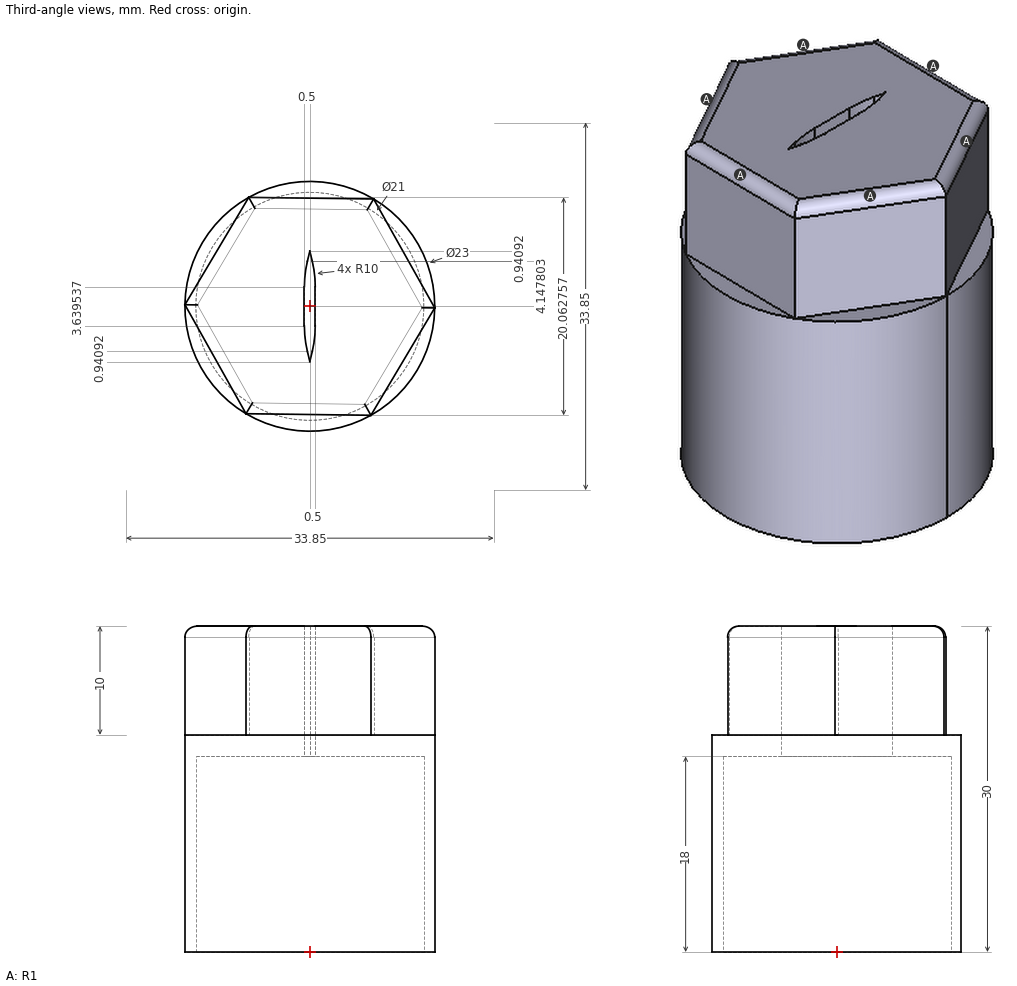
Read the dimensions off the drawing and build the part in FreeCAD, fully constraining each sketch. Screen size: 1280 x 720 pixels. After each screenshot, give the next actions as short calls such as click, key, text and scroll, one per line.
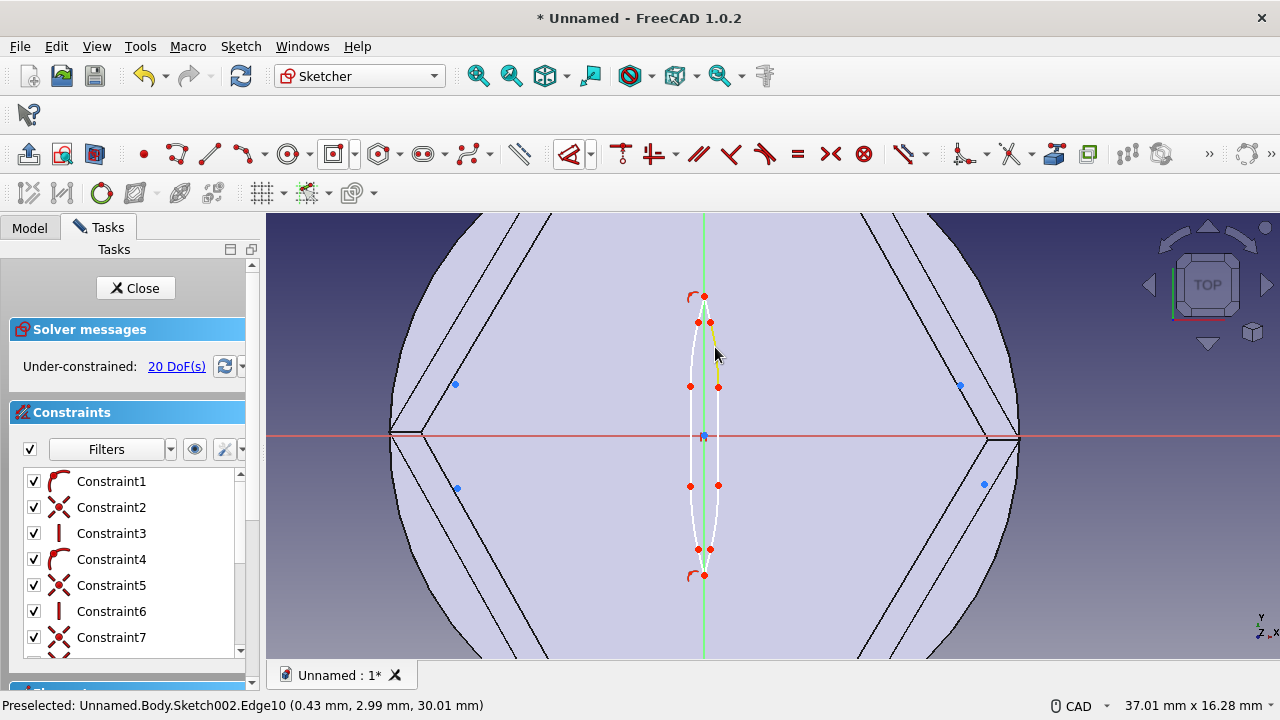
scroll(709, 315, up, 6)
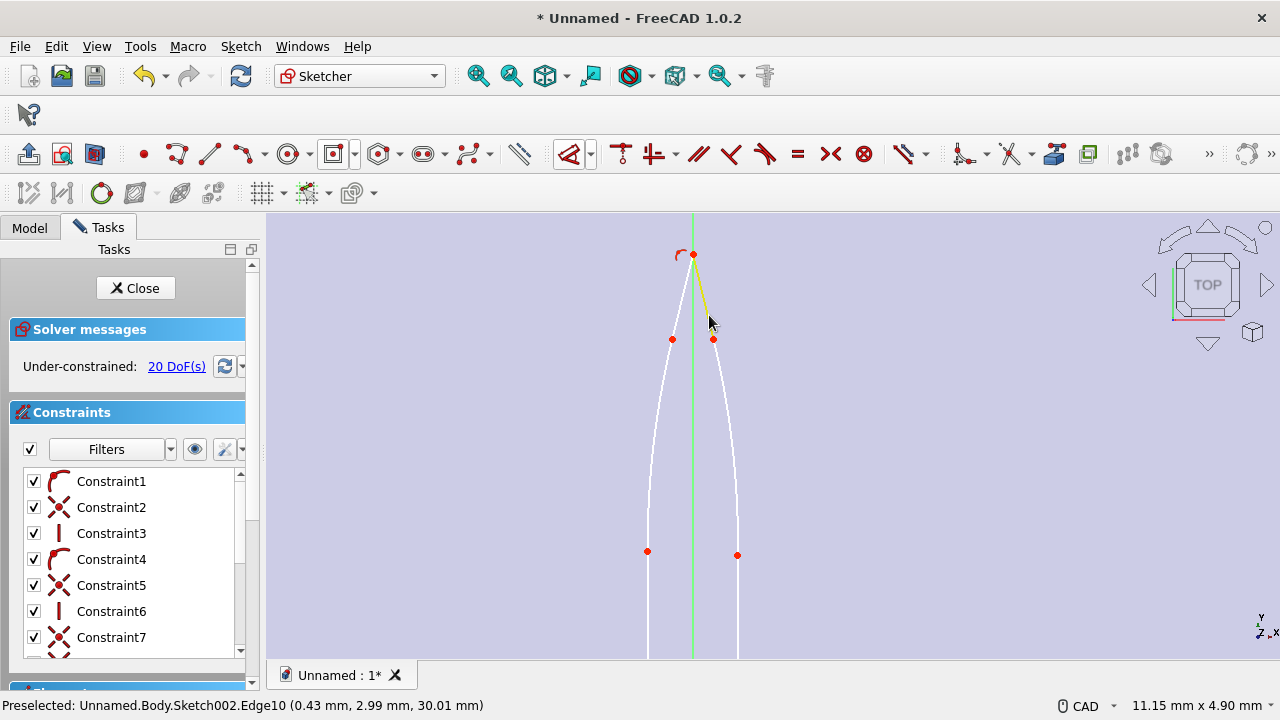
click(707, 314)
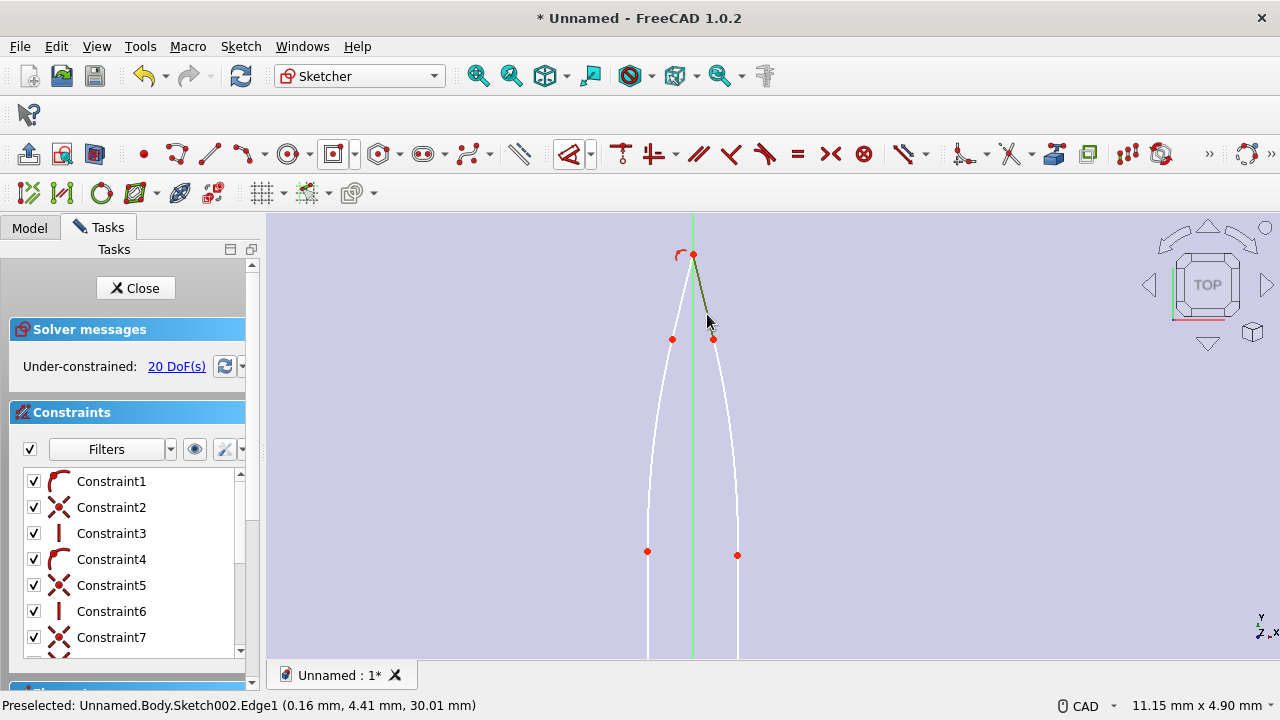
click(736, 490)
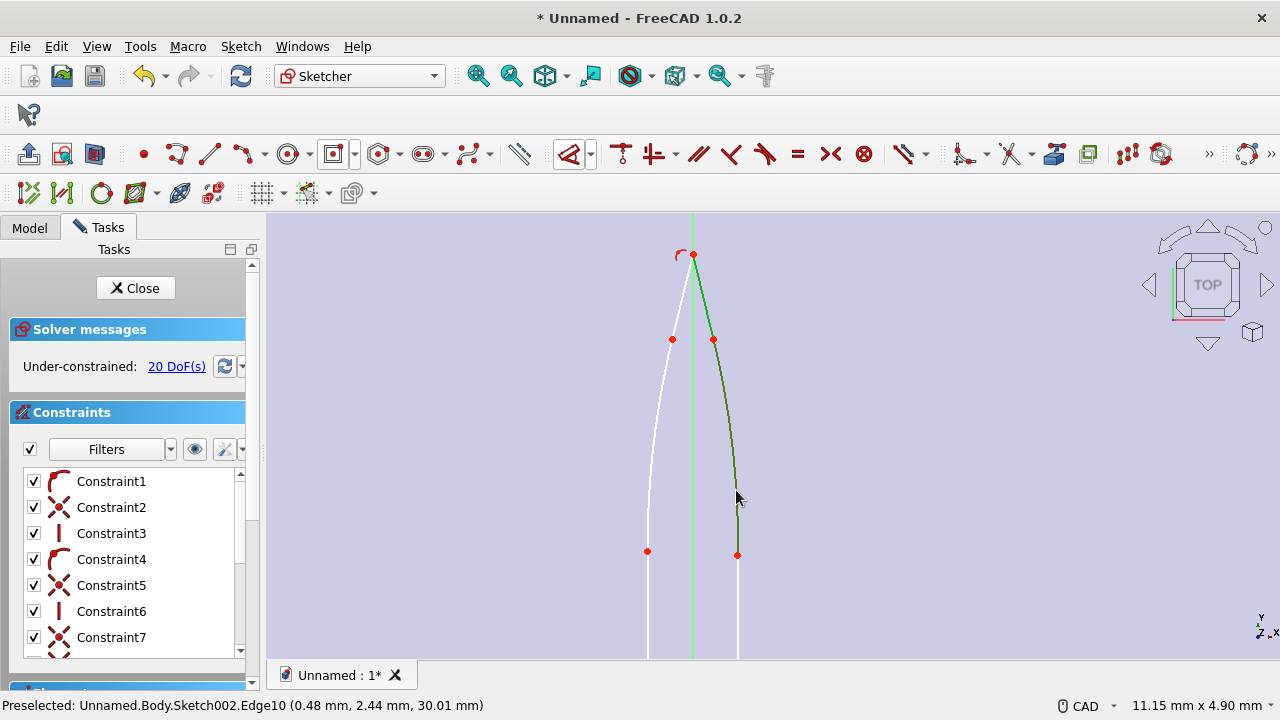
click(765, 154)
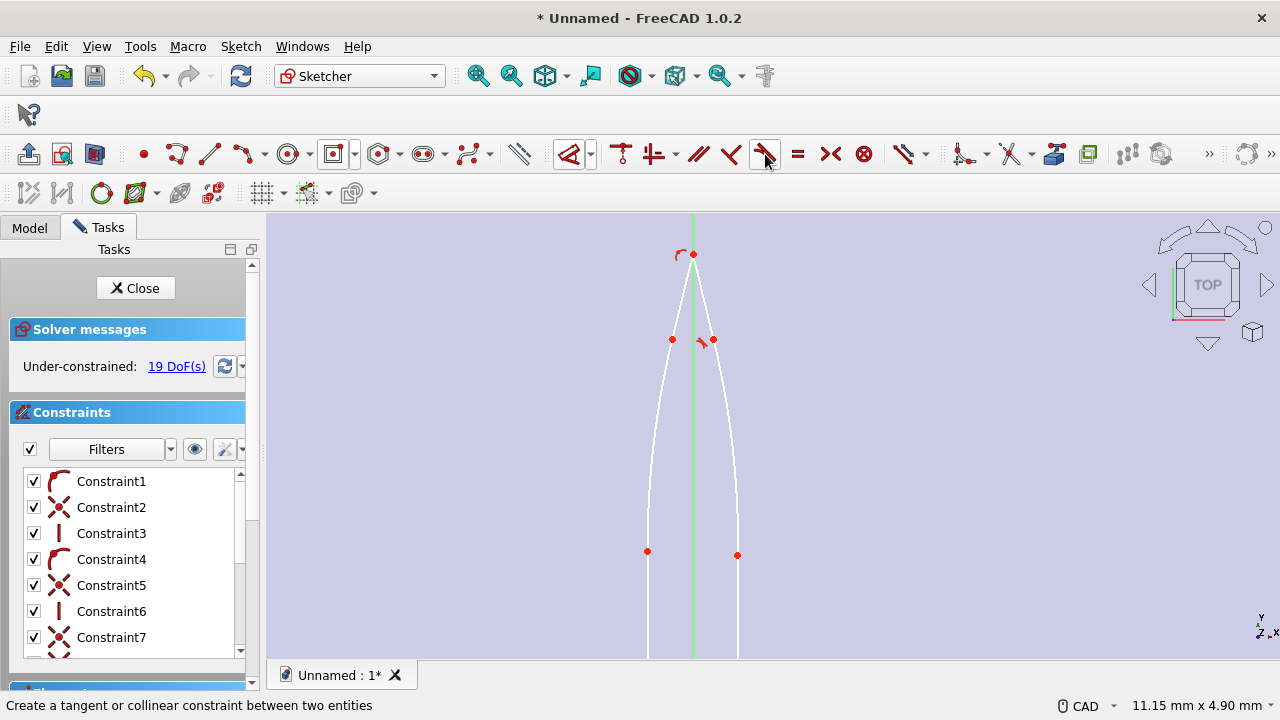
click(678, 314)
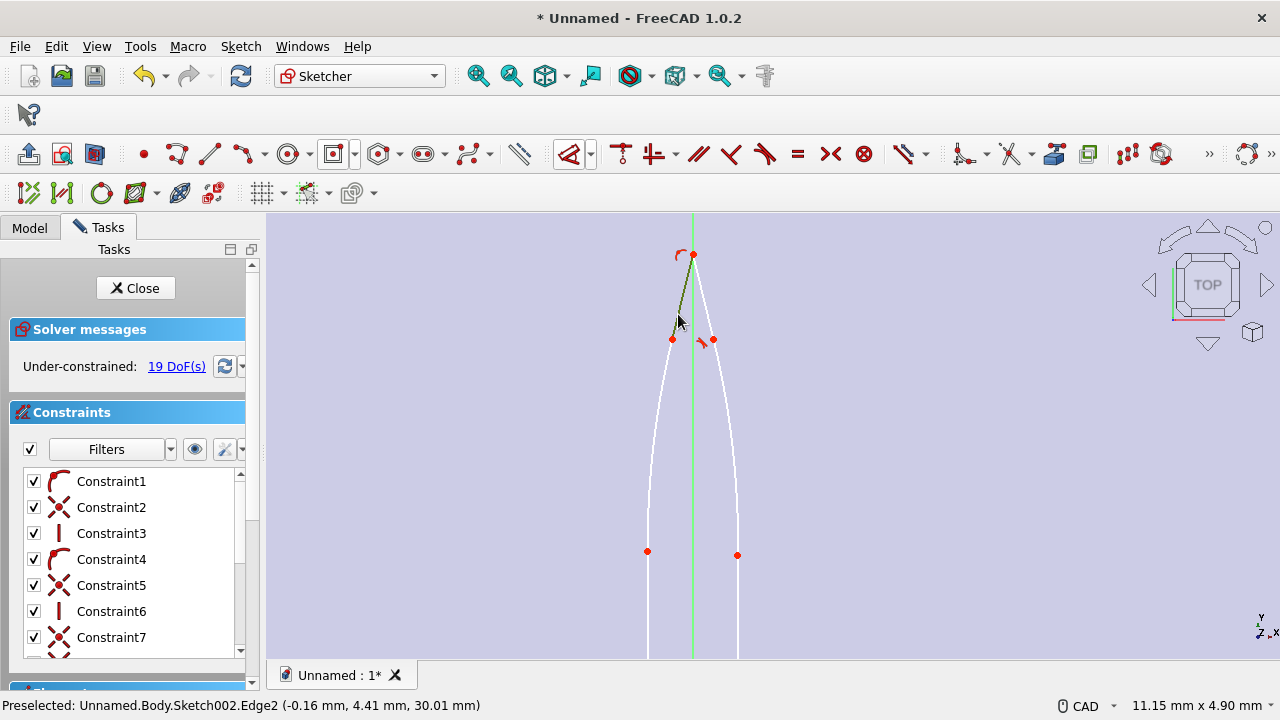
click(659, 403)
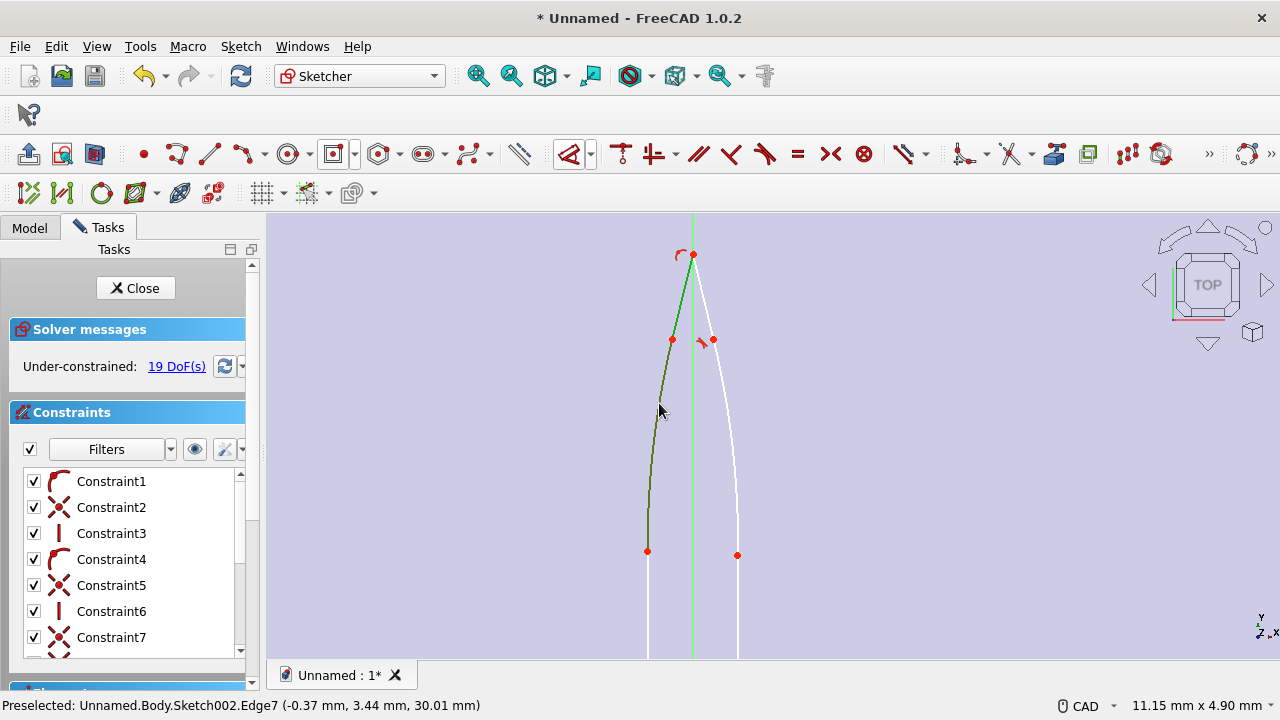
click(765, 154)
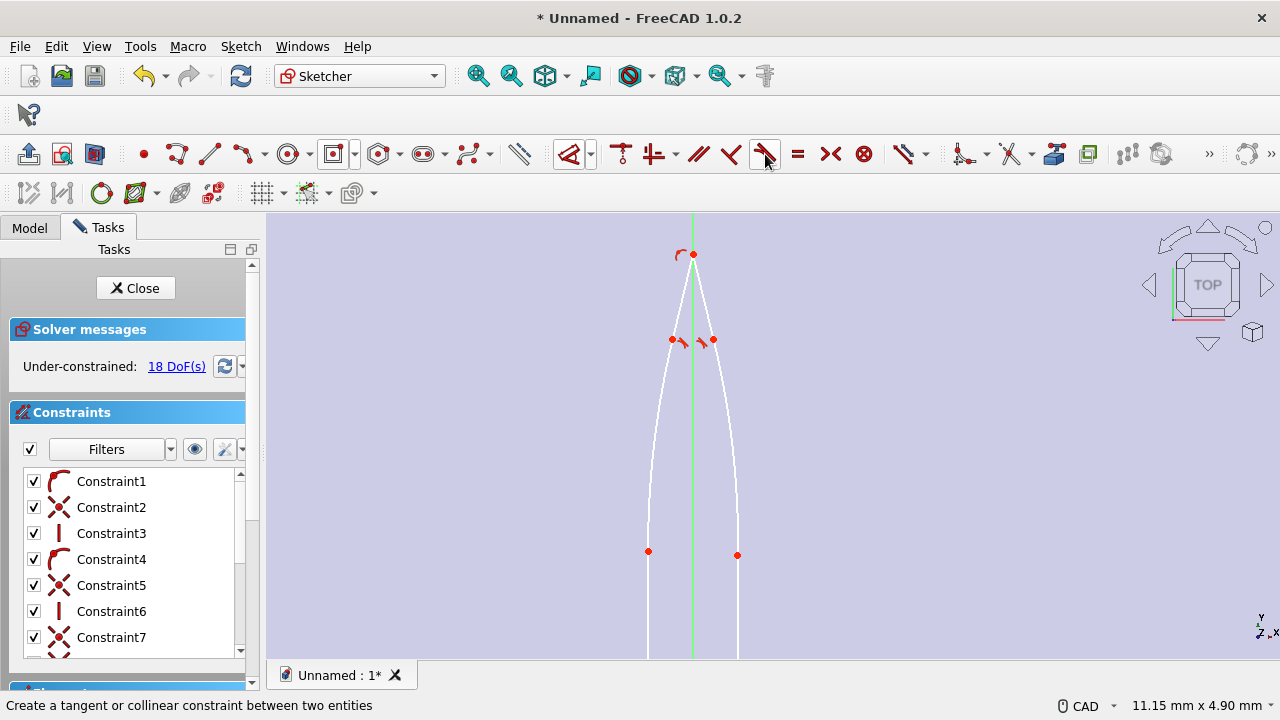
click(648, 618)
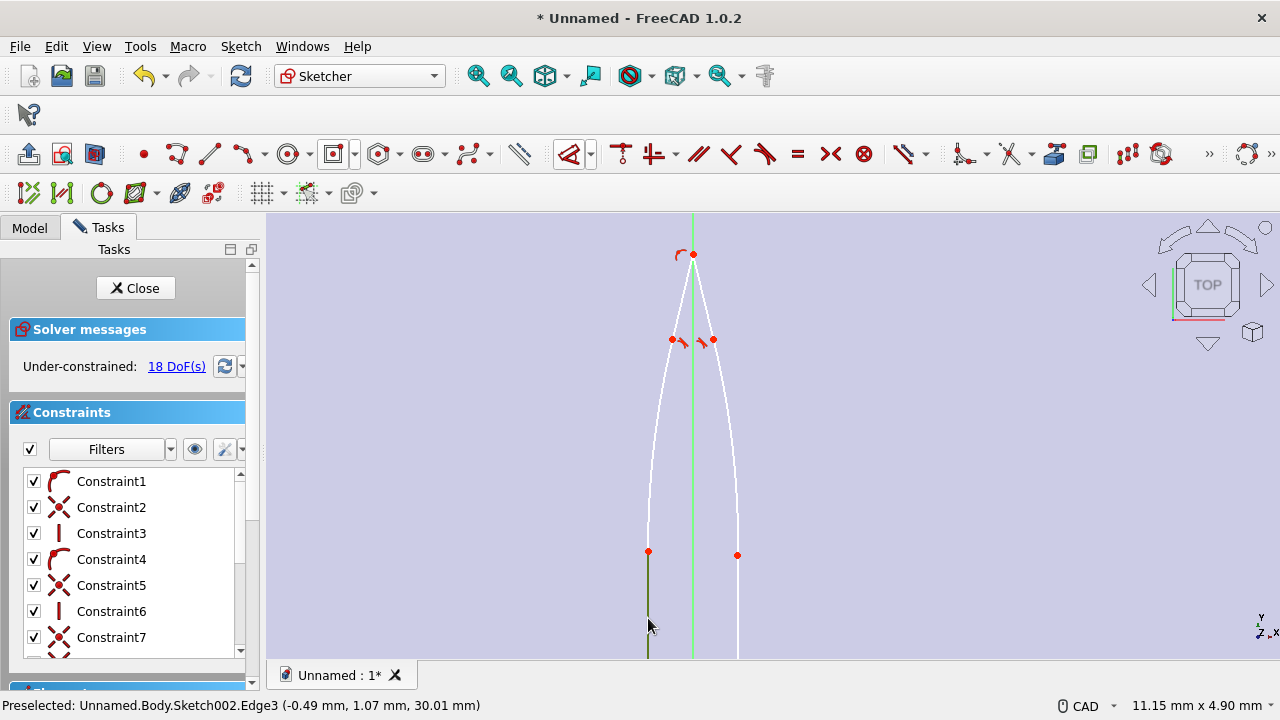
click(660, 403)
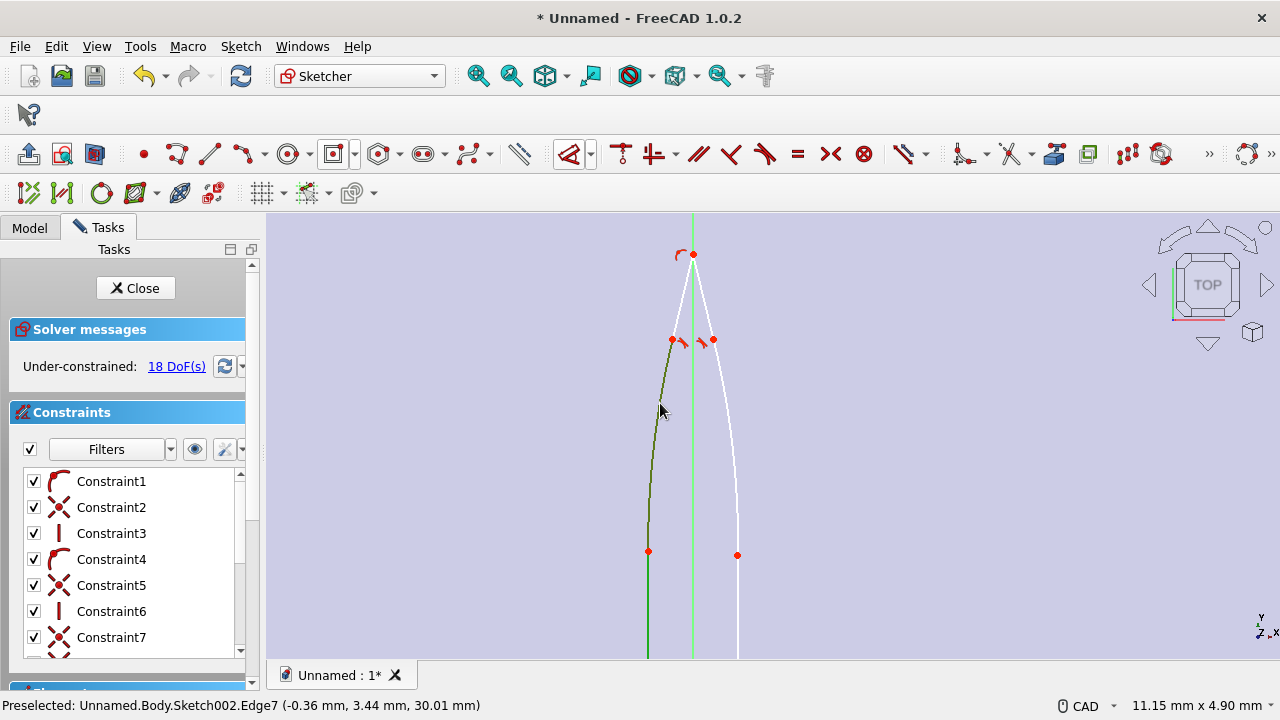
key(t)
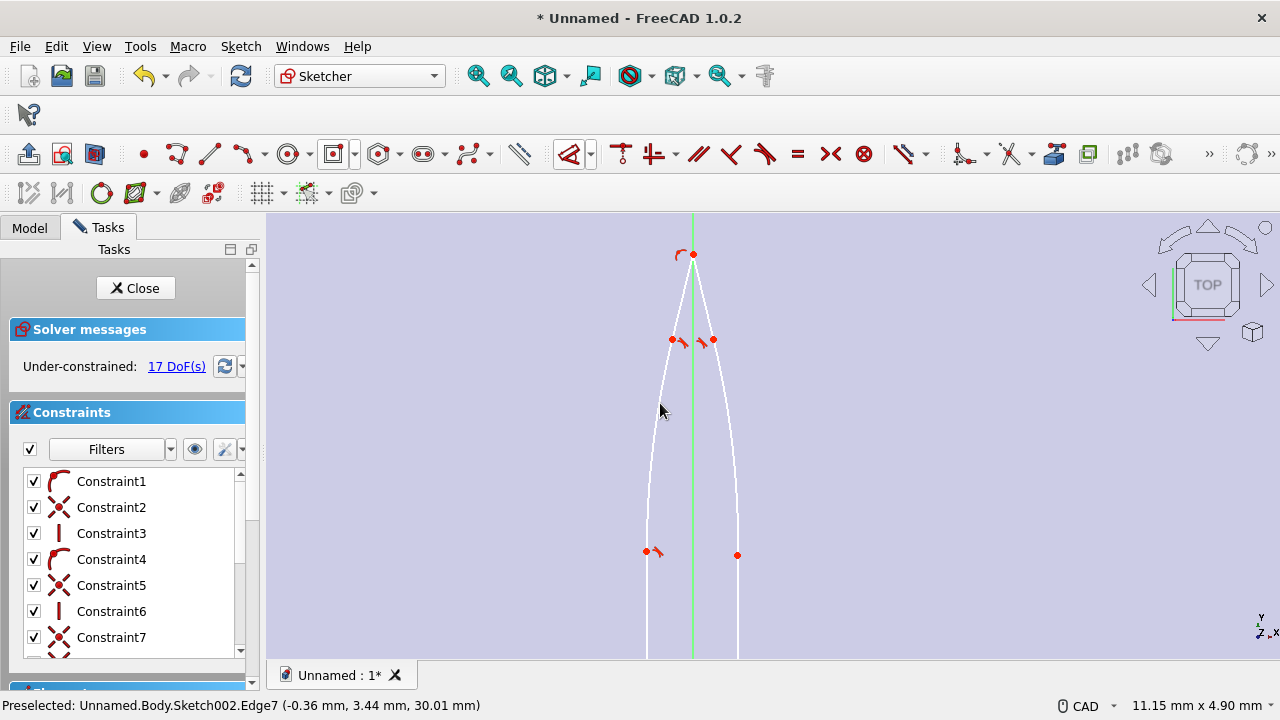
click(647, 618)